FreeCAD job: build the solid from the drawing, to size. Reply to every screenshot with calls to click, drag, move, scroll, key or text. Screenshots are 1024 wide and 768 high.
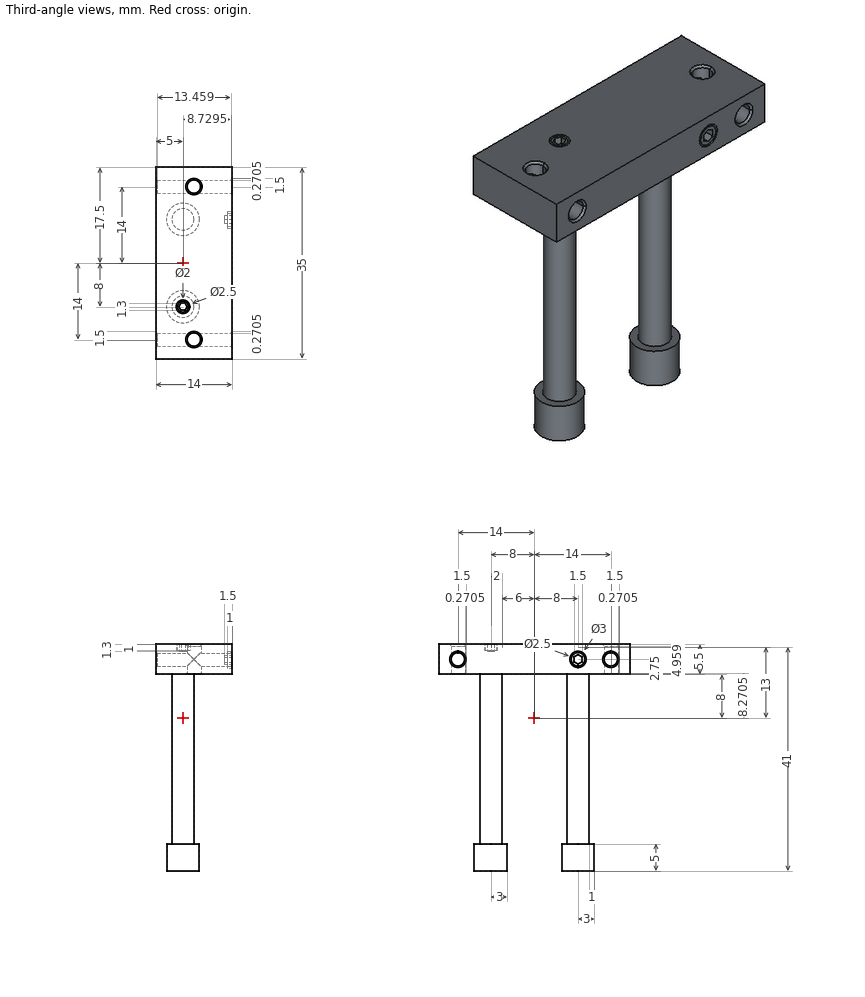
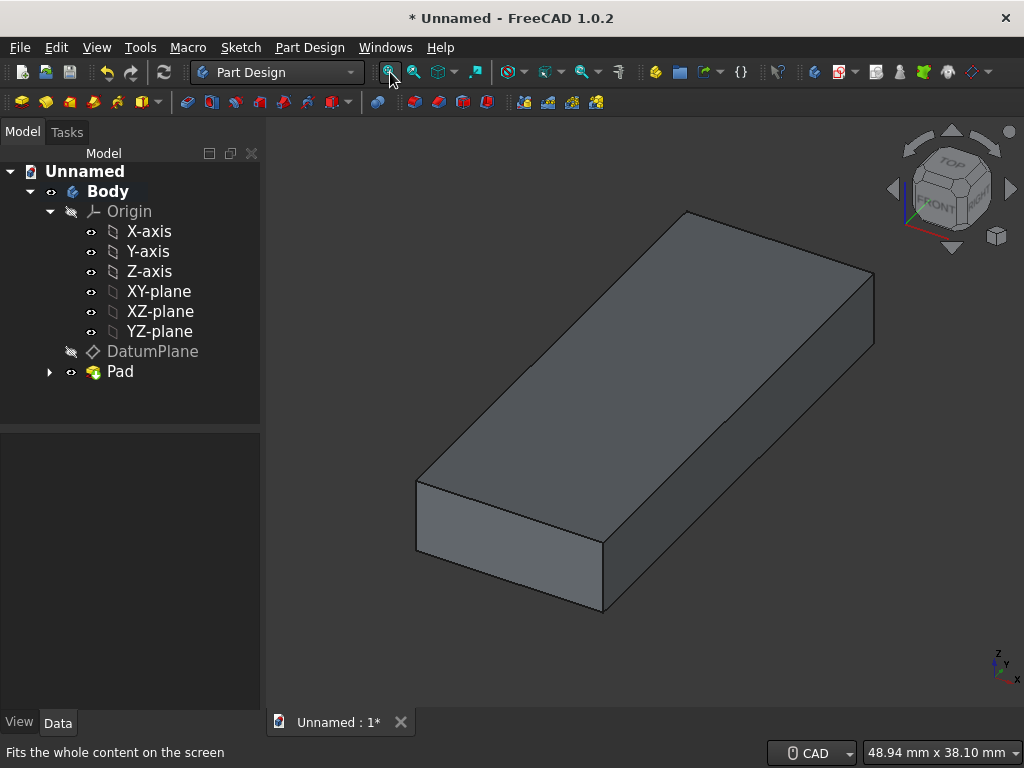
click(840, 72)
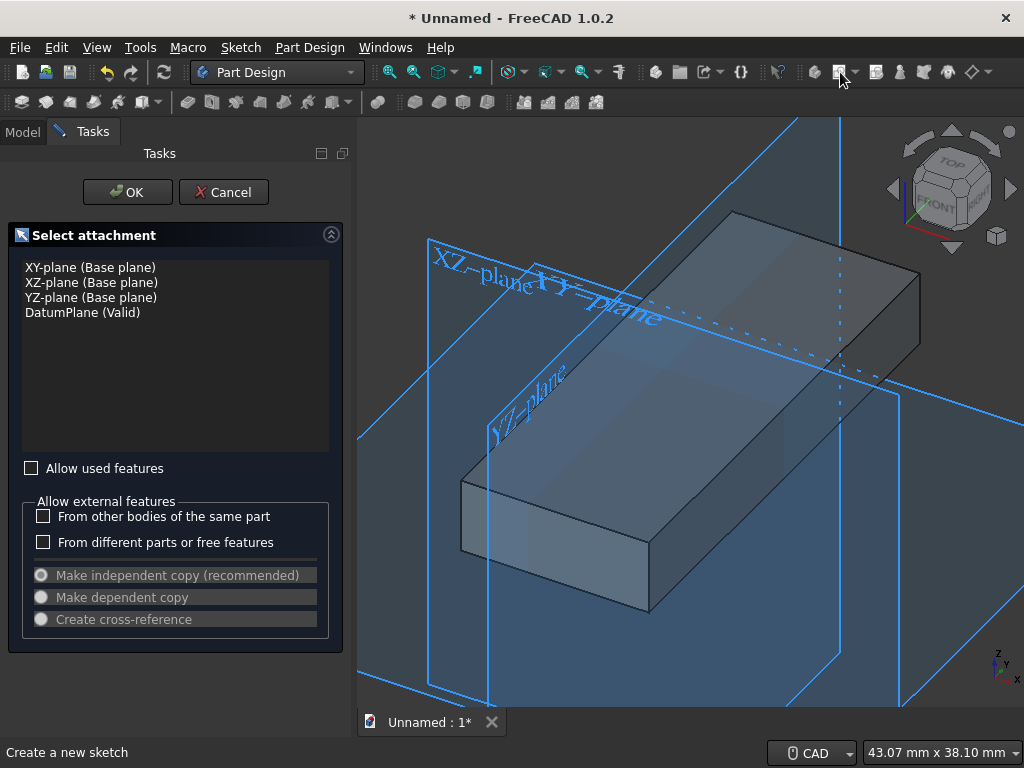
click(82, 298)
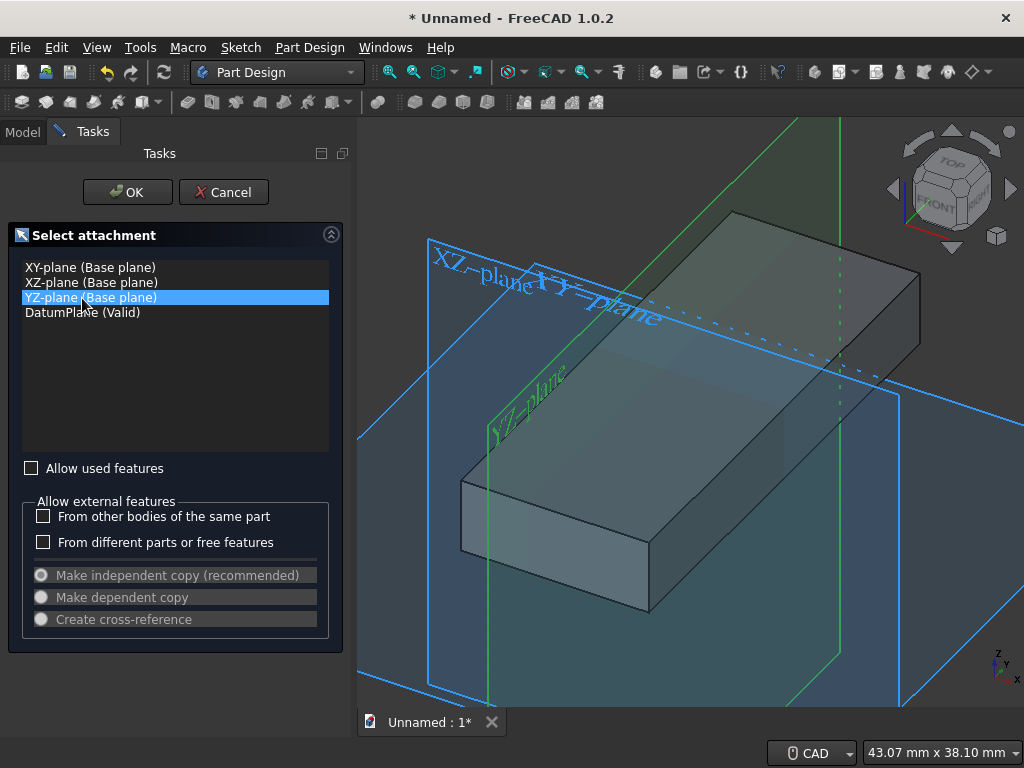
click(128, 192)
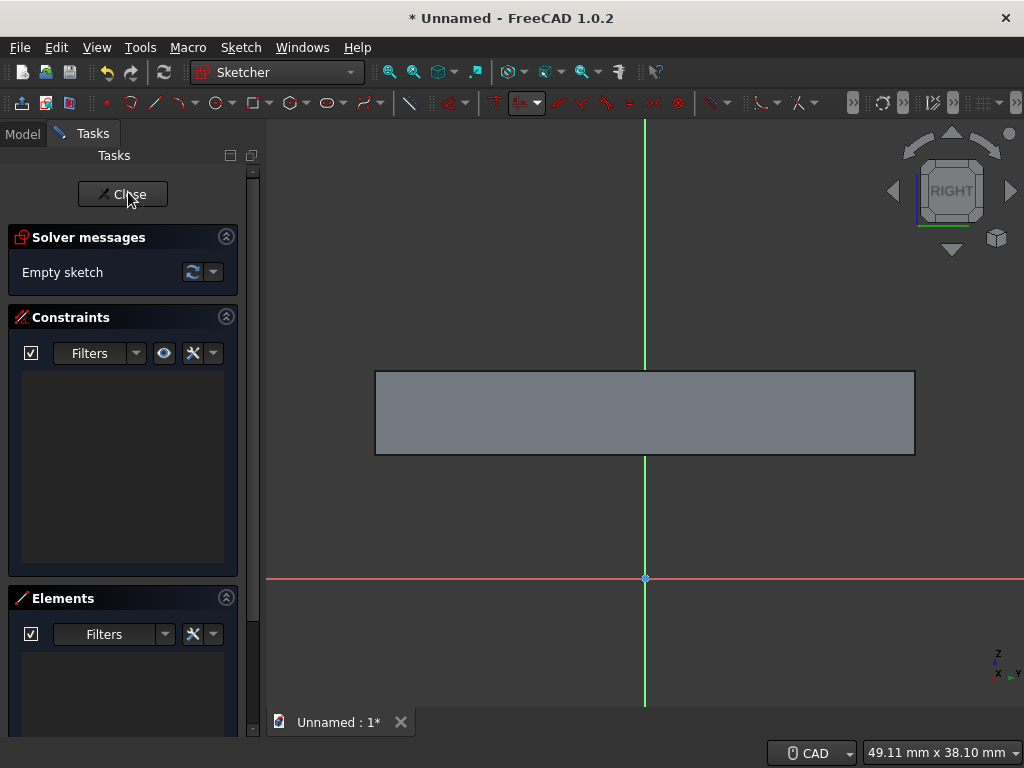
click(70, 104)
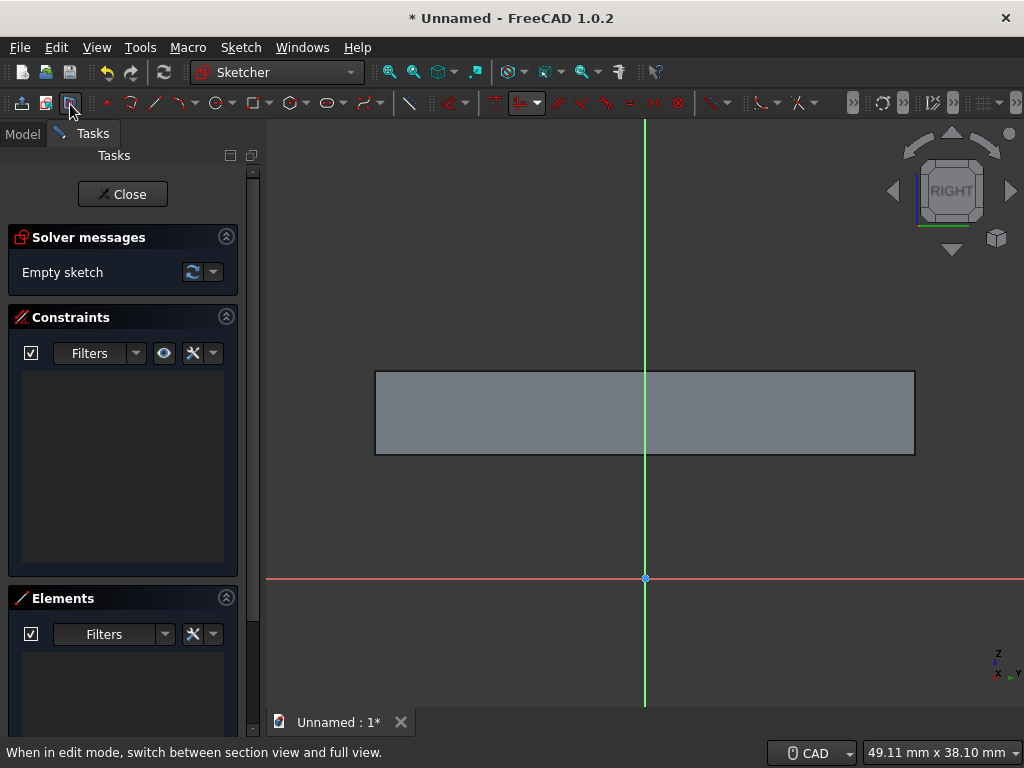
scroll(451, 286, down, 4)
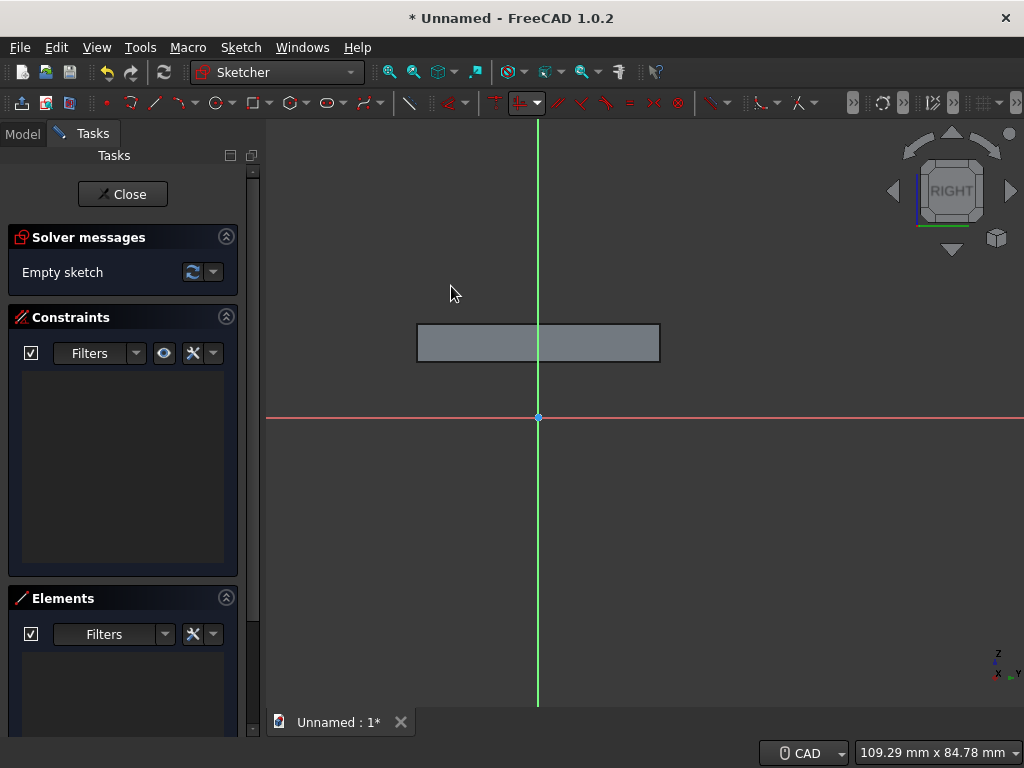
click(132, 104)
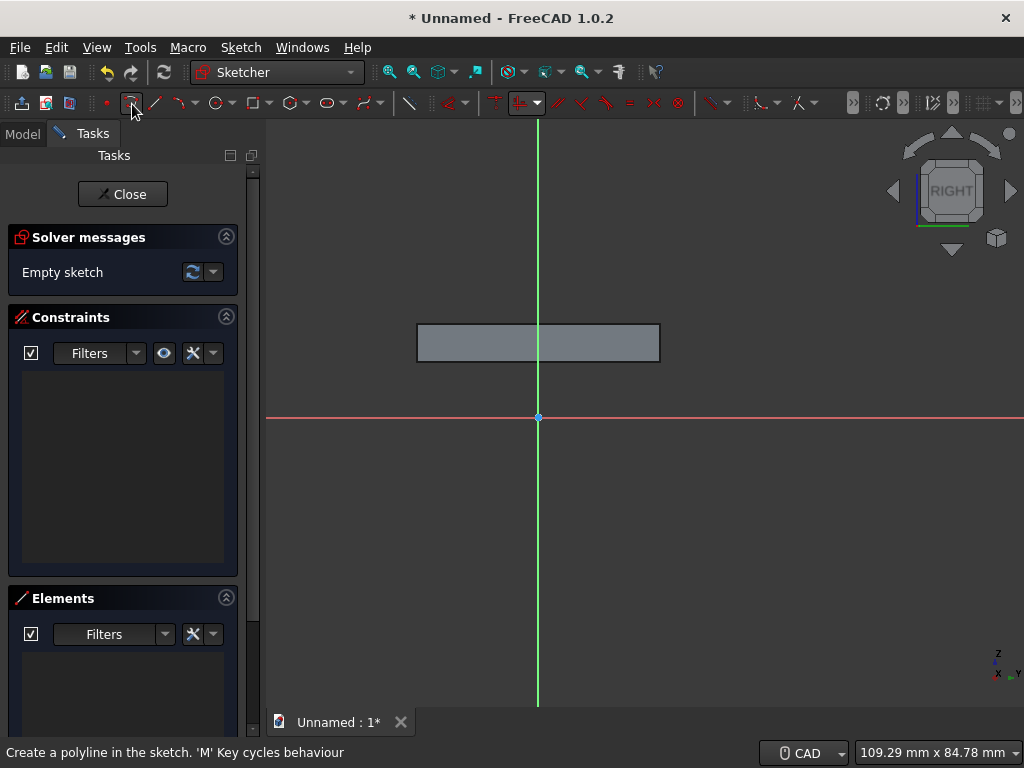
click(594, 328)
click(594, 612)
click(615, 612)
click(615, 577)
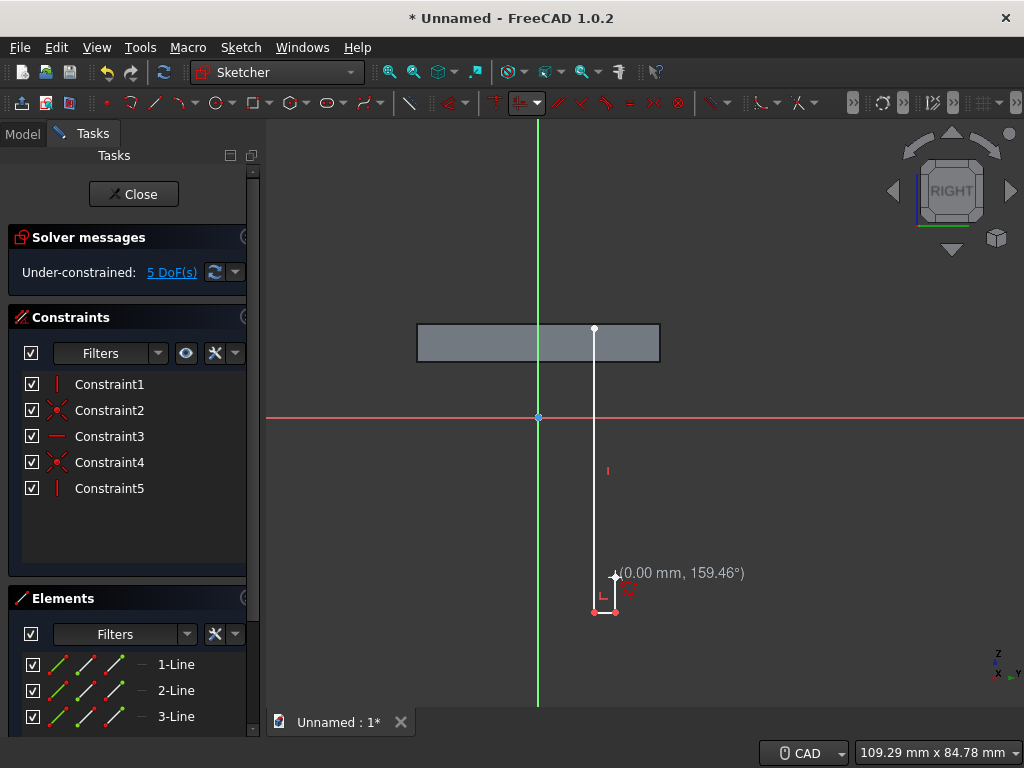
scroll(608, 577, up, 5)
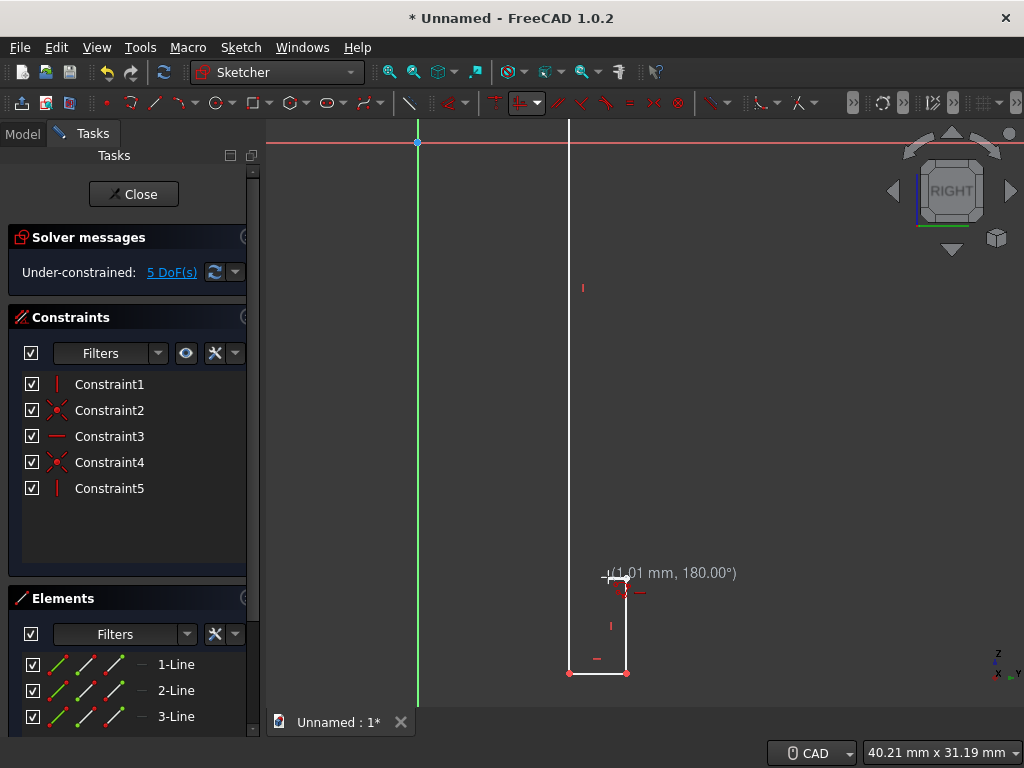
click(606, 576)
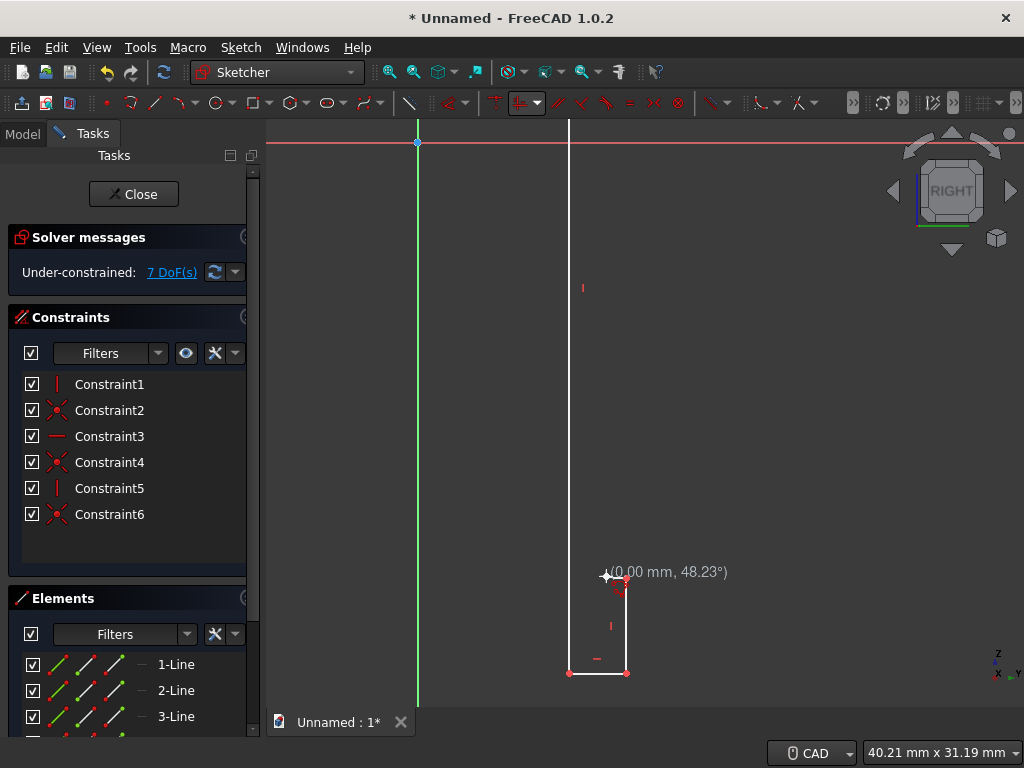
scroll(609, 578, down, 5)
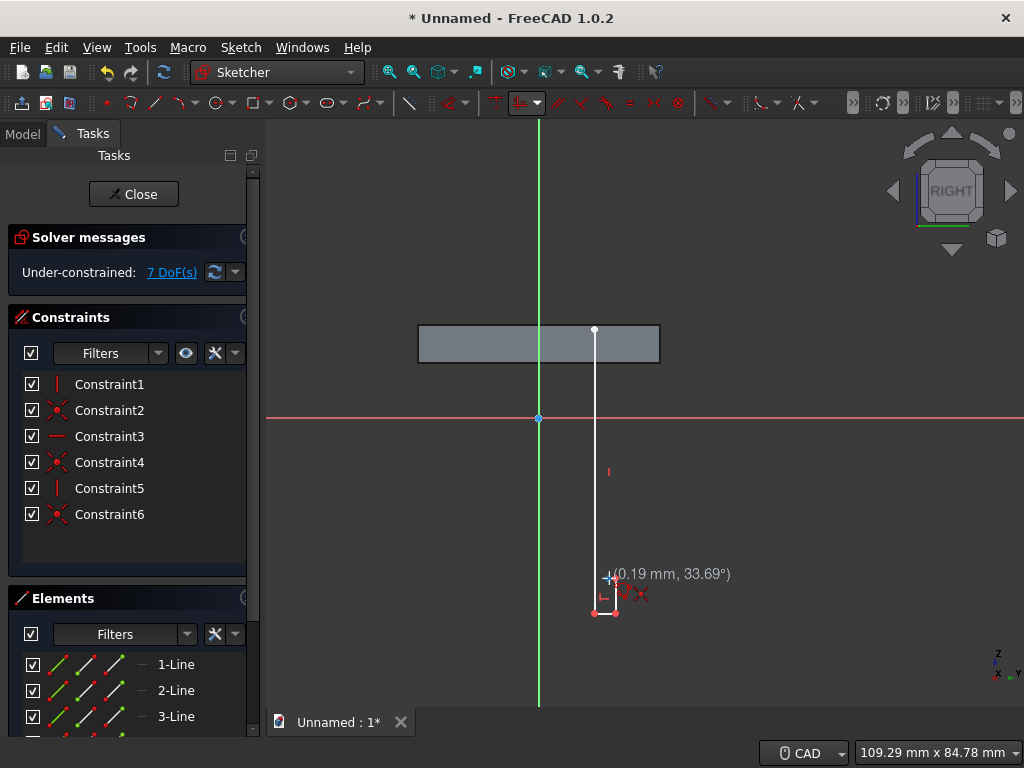
click(608, 328)
click(595, 330)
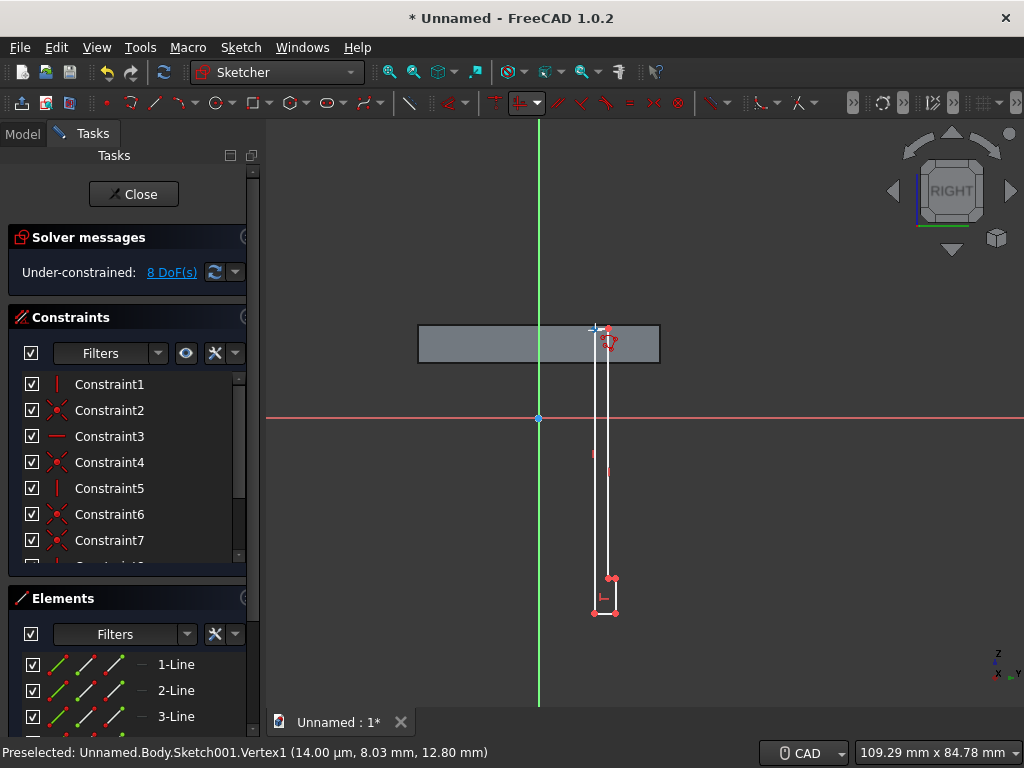
click(156, 104)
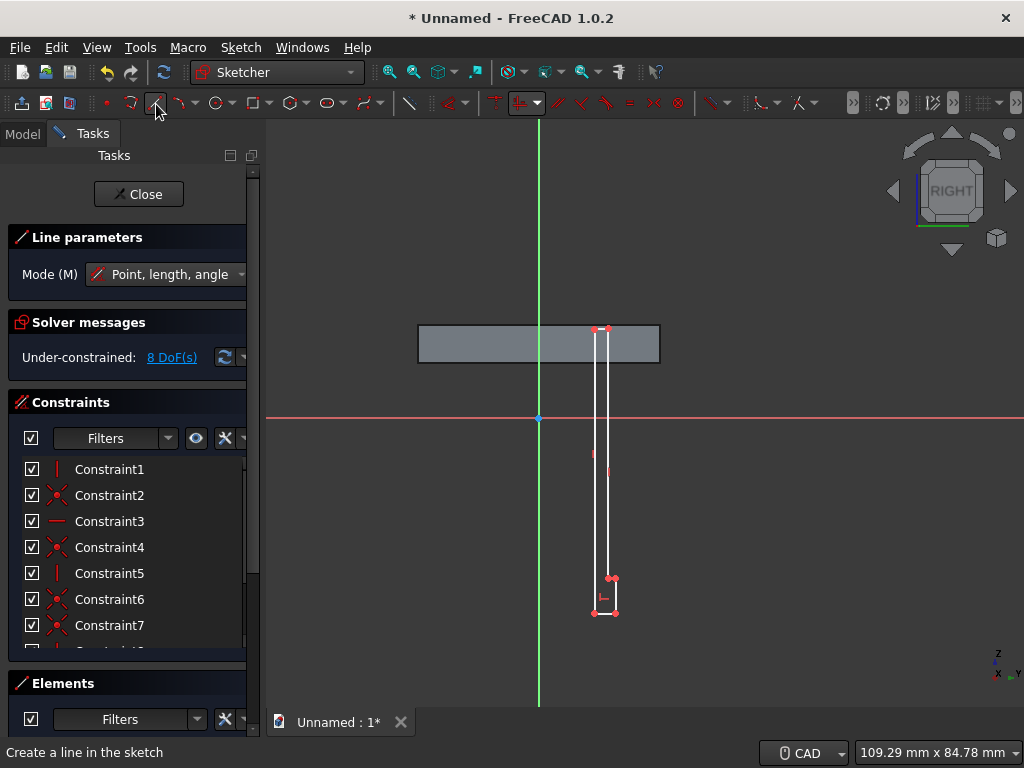
click(594, 300)
click(594, 215)
key(Escape)